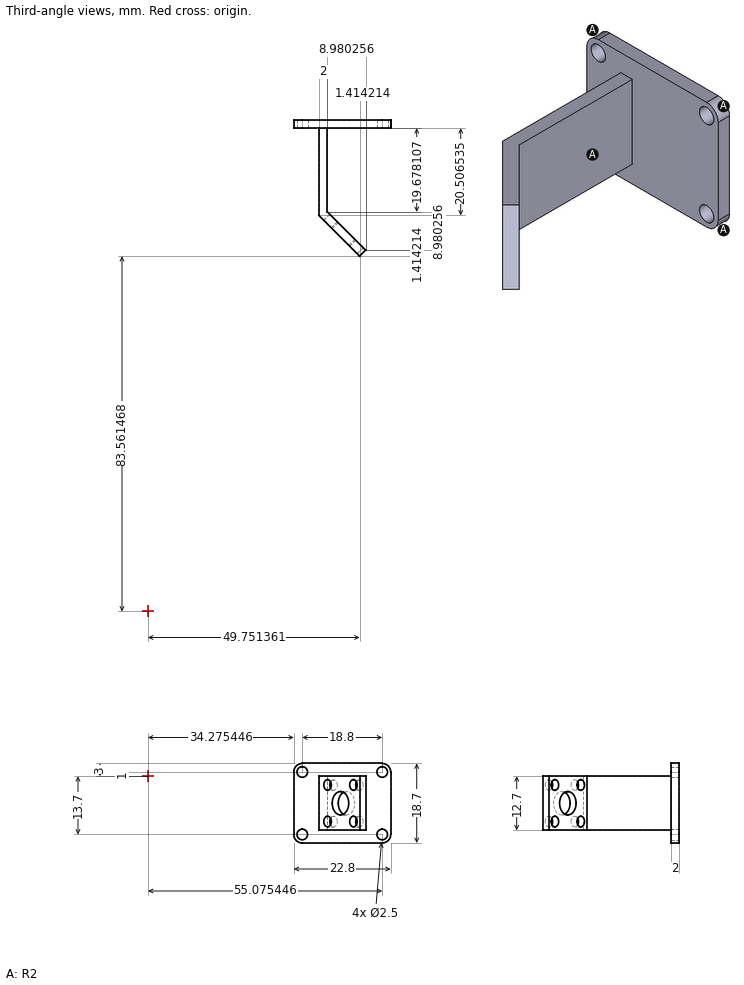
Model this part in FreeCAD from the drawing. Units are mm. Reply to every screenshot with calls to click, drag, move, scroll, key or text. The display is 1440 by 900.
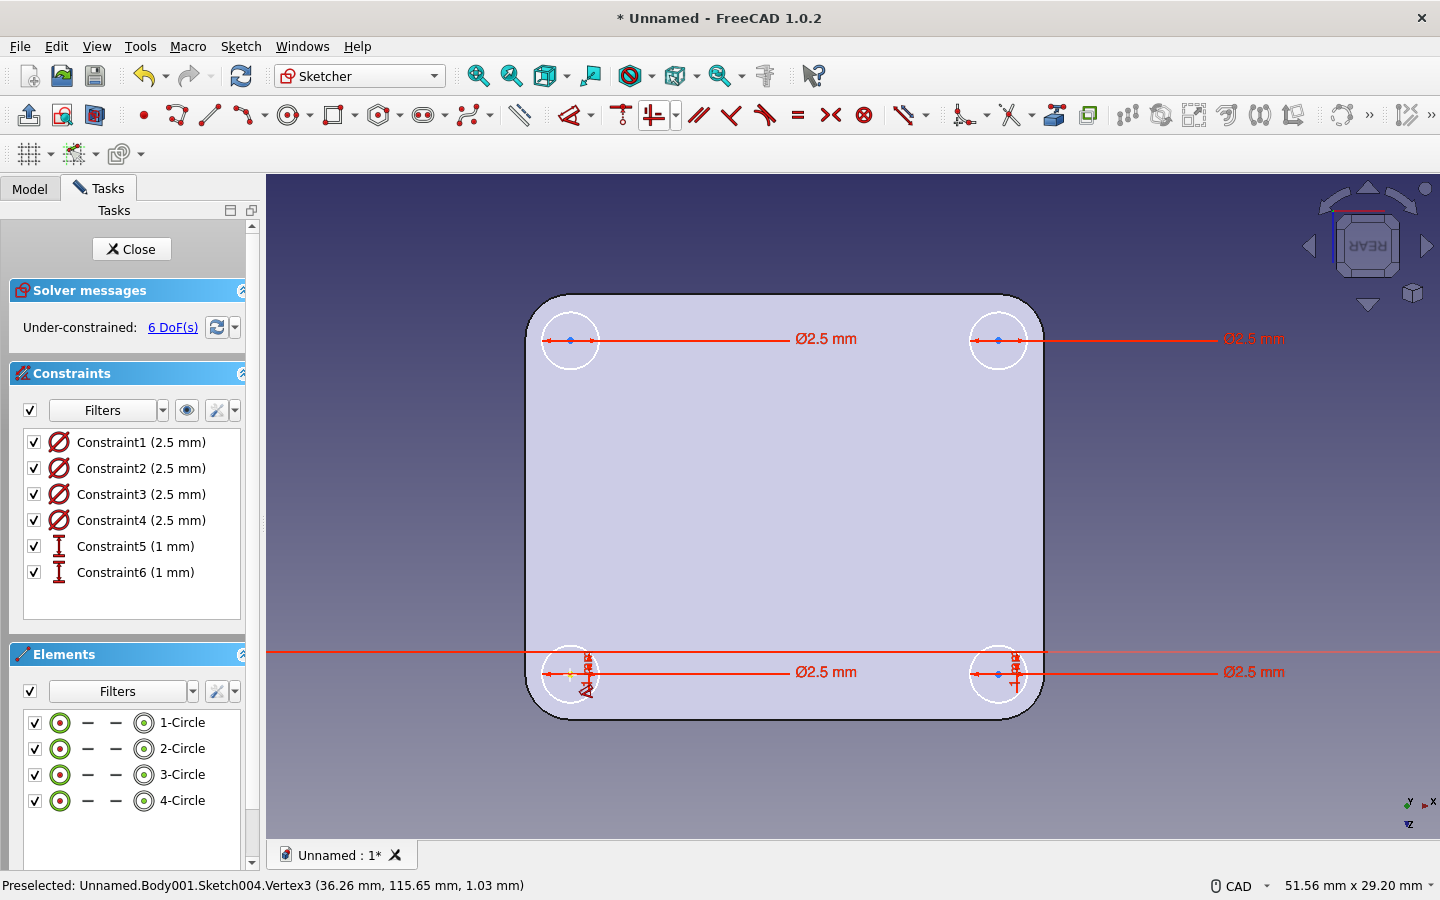
click(998, 341)
click(1032, 496)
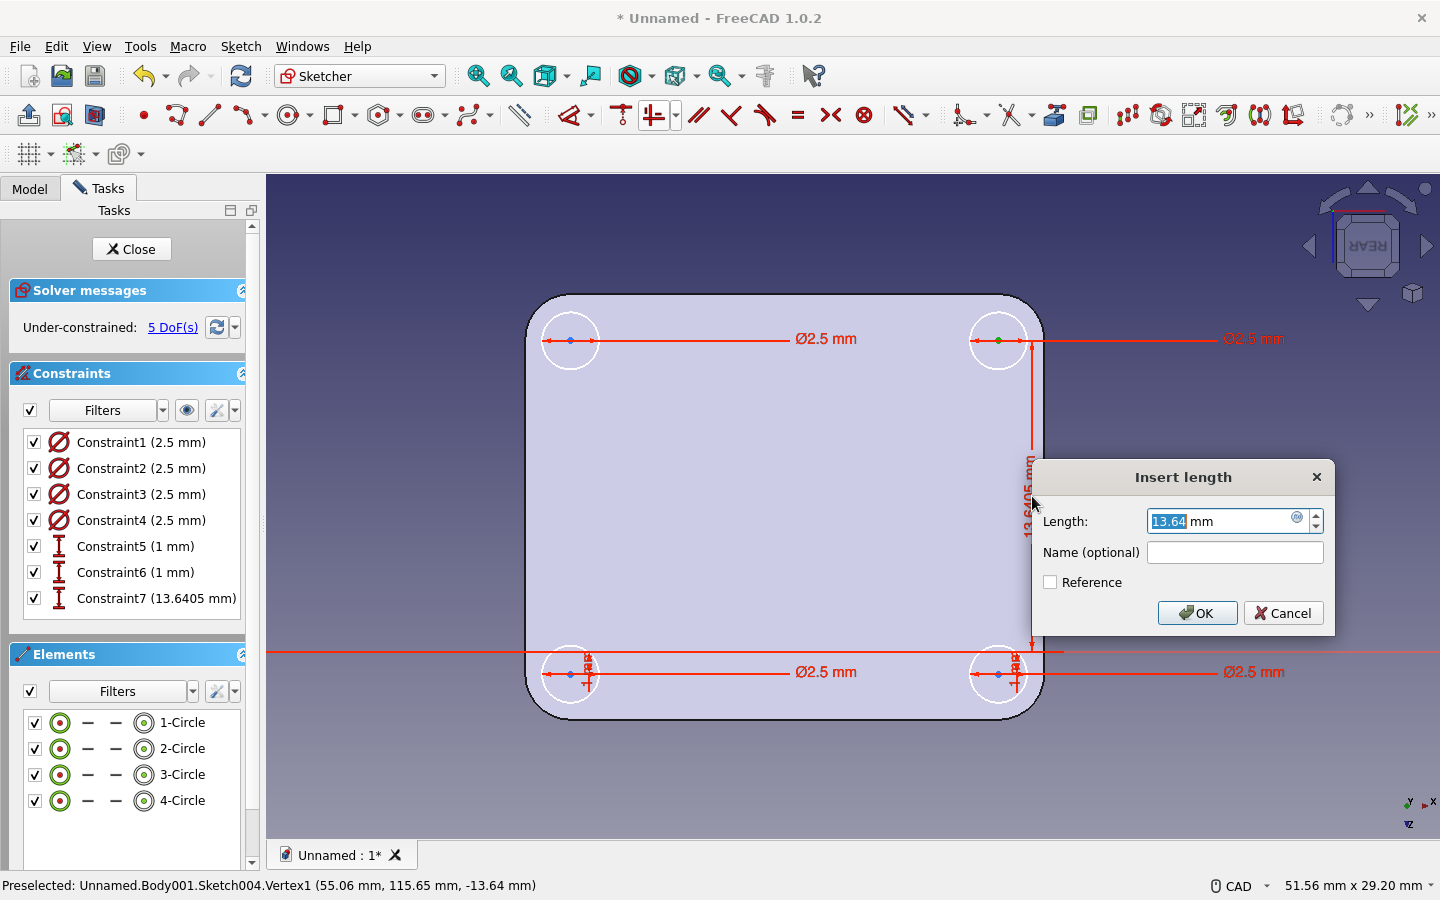
text(13.7)
key(Return)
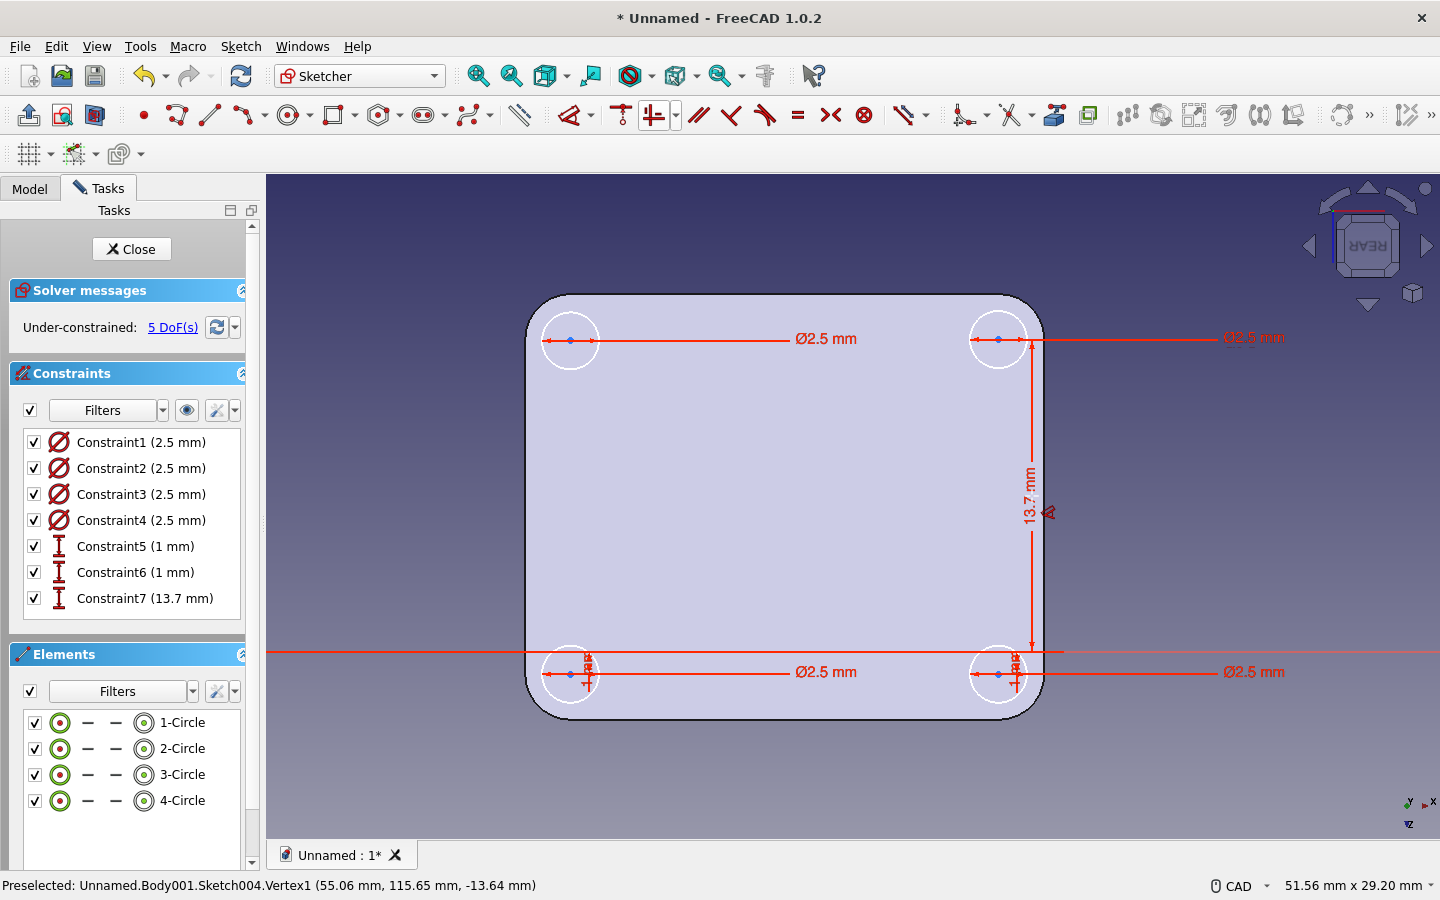
click(570, 341)
click(604, 496)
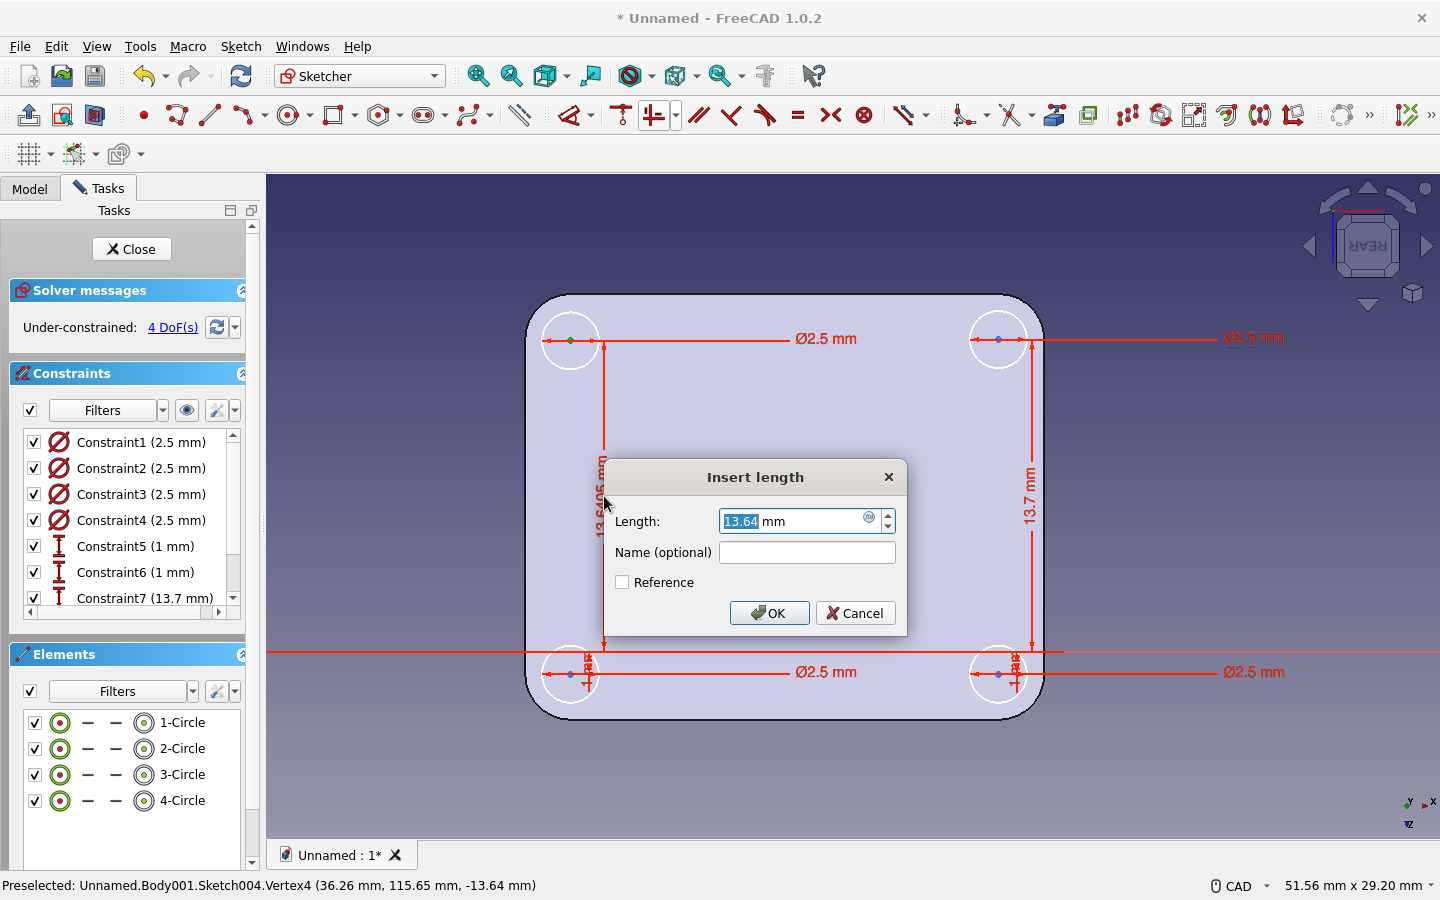
text(13.7)
key(Return)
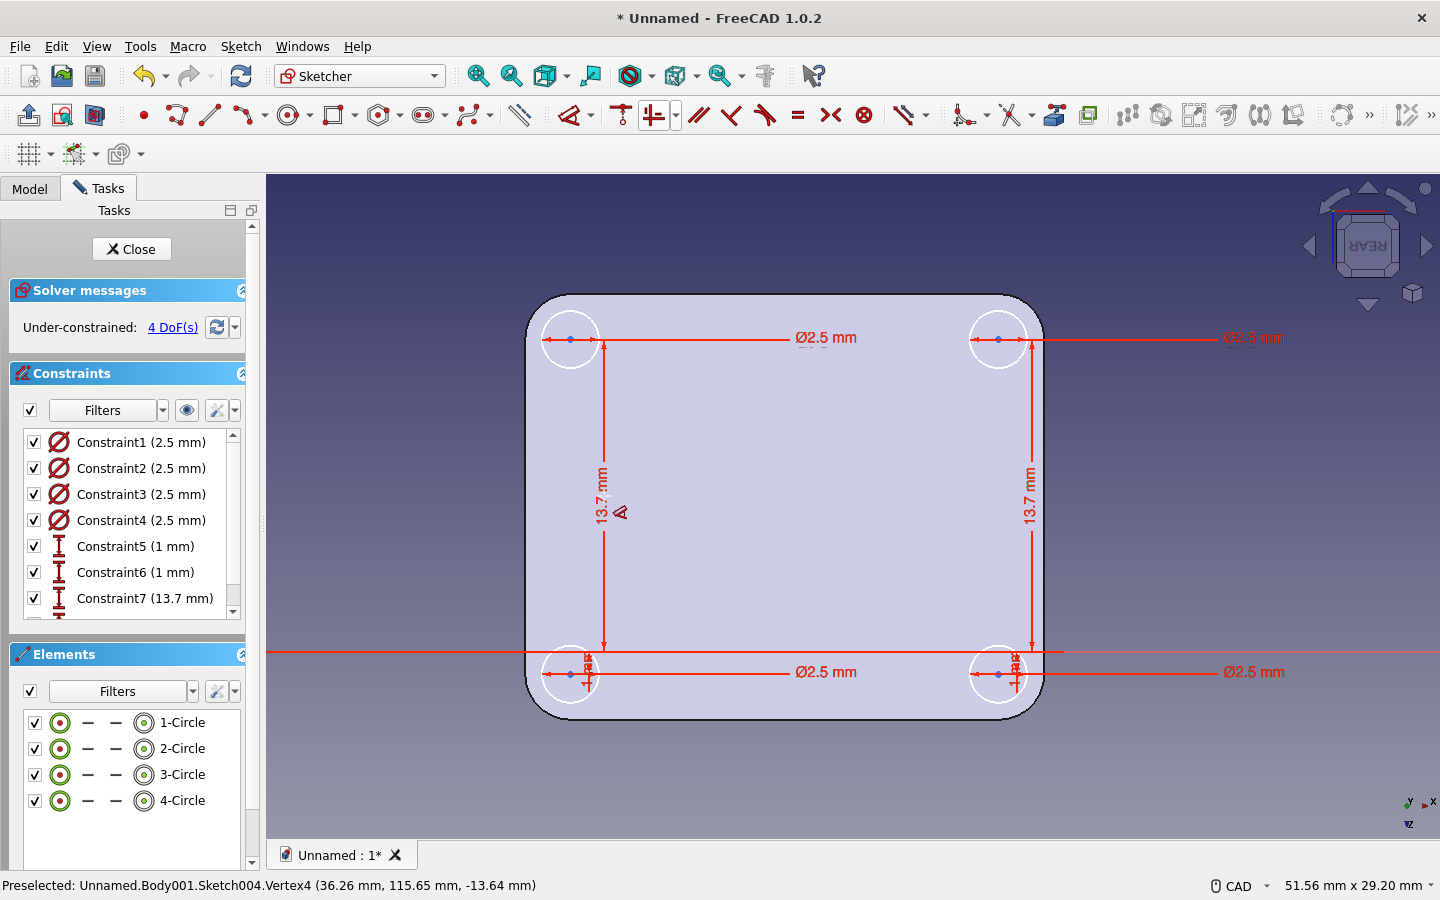
click(998, 674)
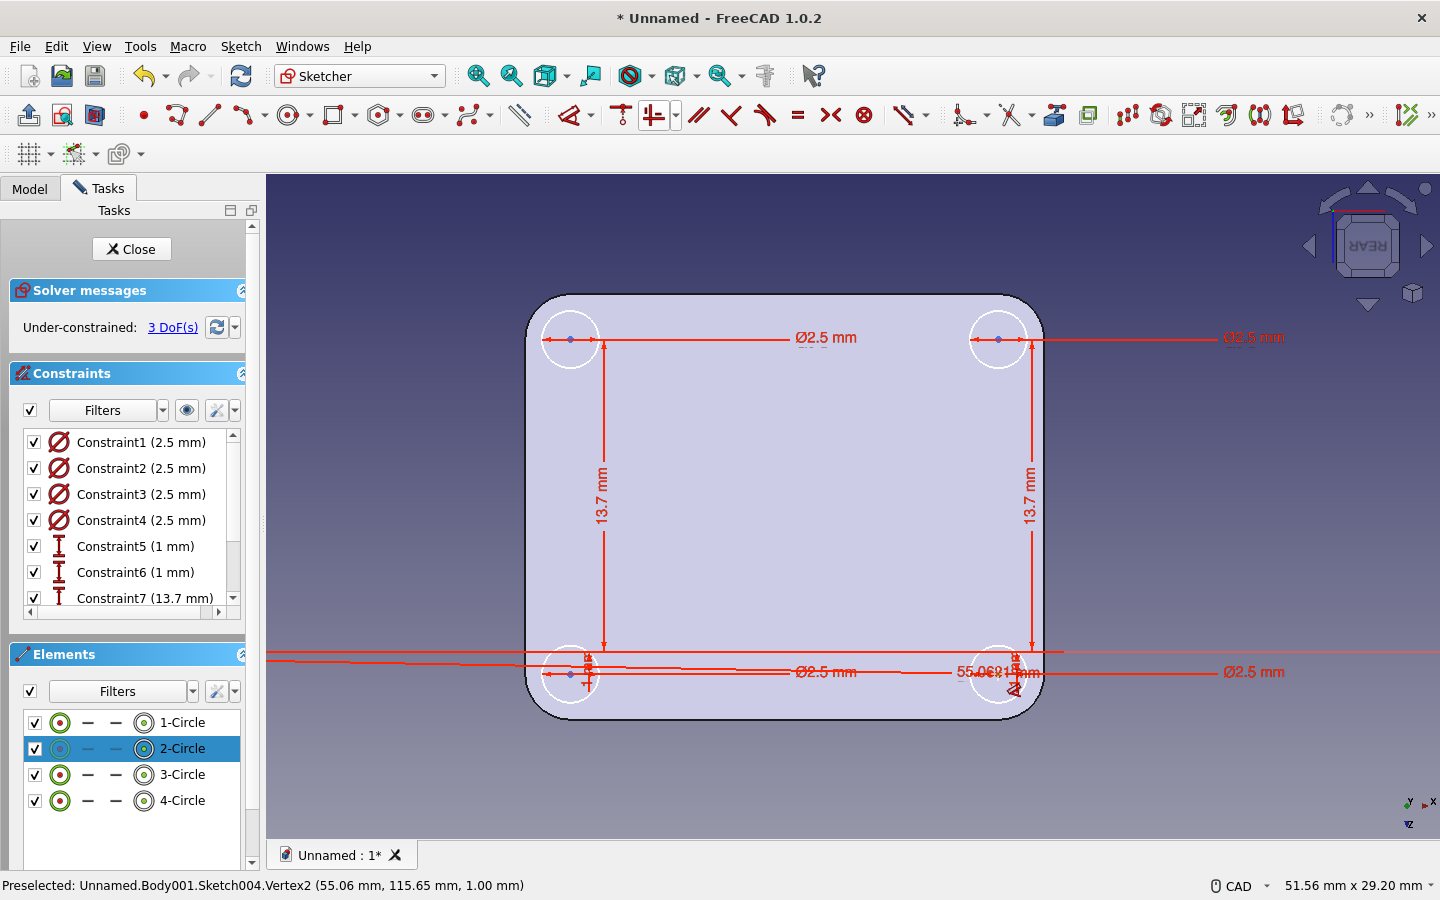
click(570, 674)
click(784, 708)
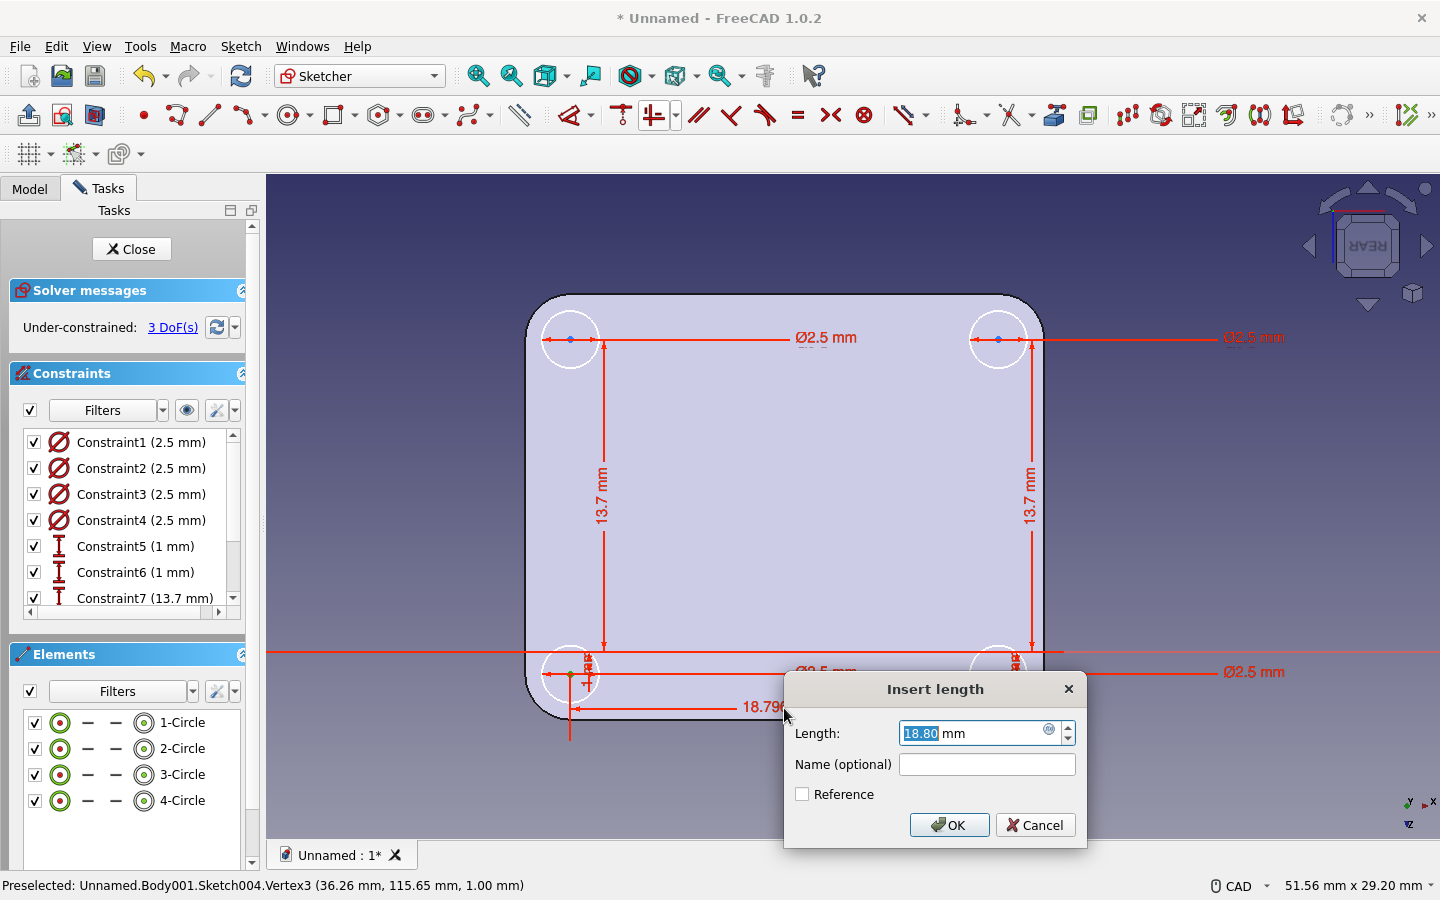
text(18.8)
key(Return)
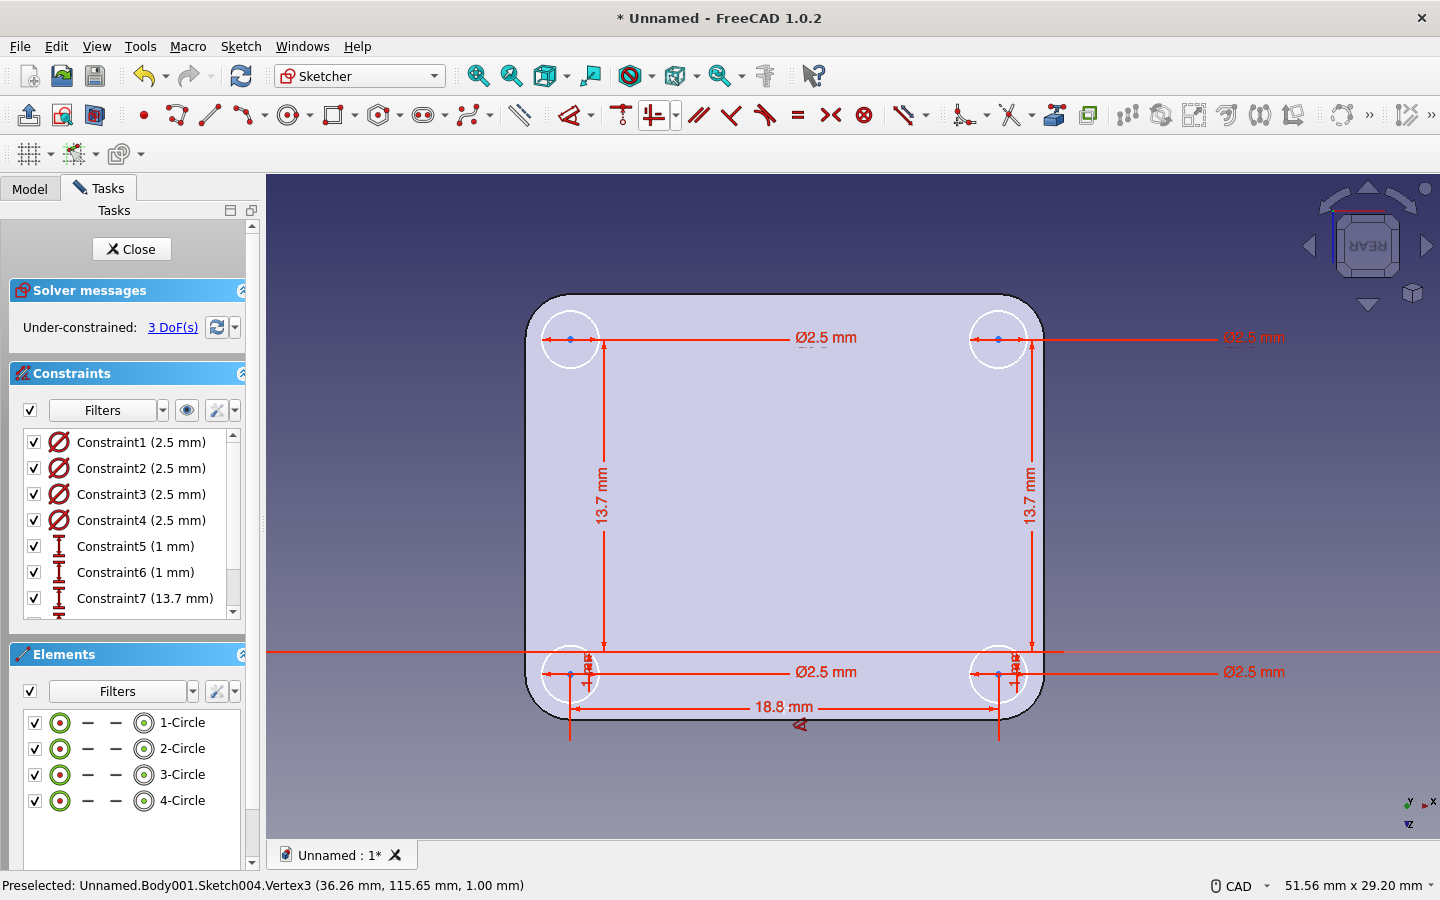
click(998, 340)